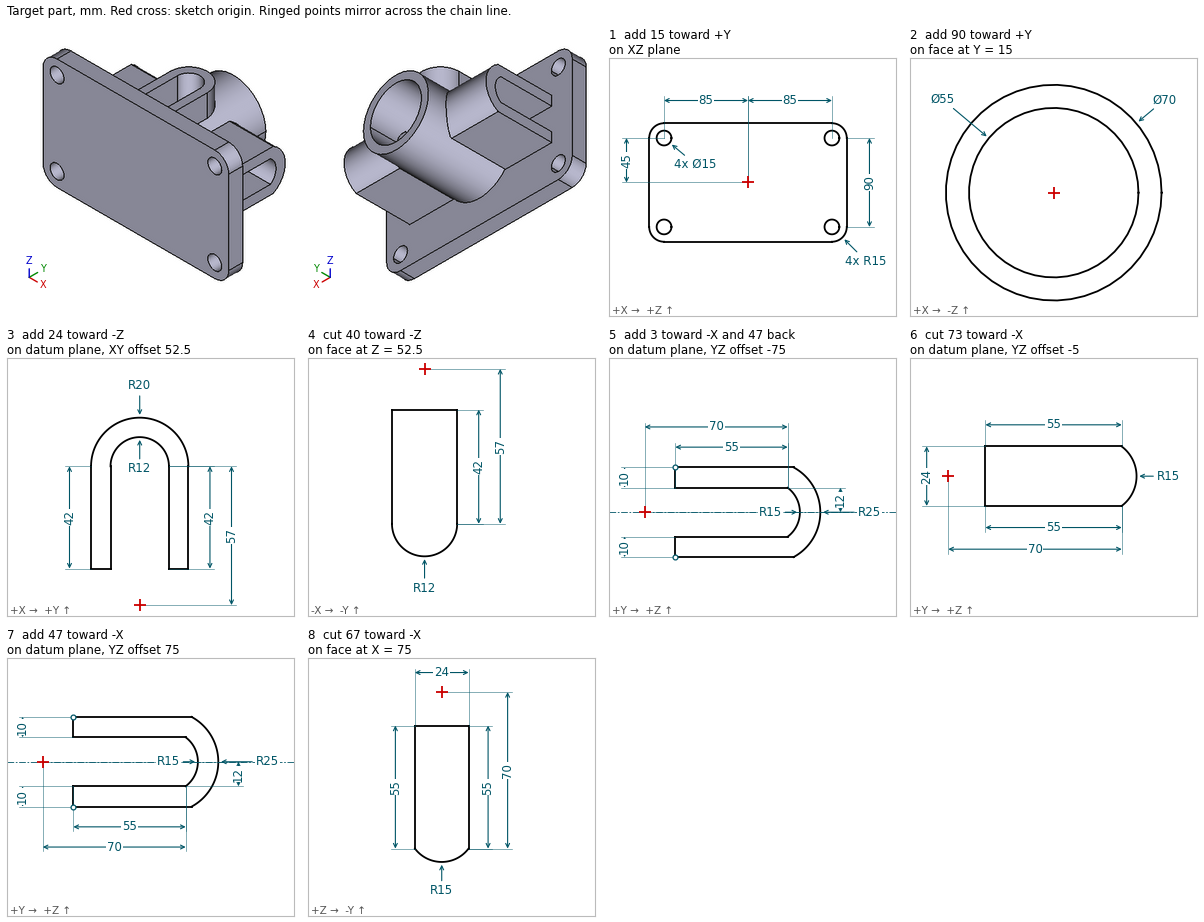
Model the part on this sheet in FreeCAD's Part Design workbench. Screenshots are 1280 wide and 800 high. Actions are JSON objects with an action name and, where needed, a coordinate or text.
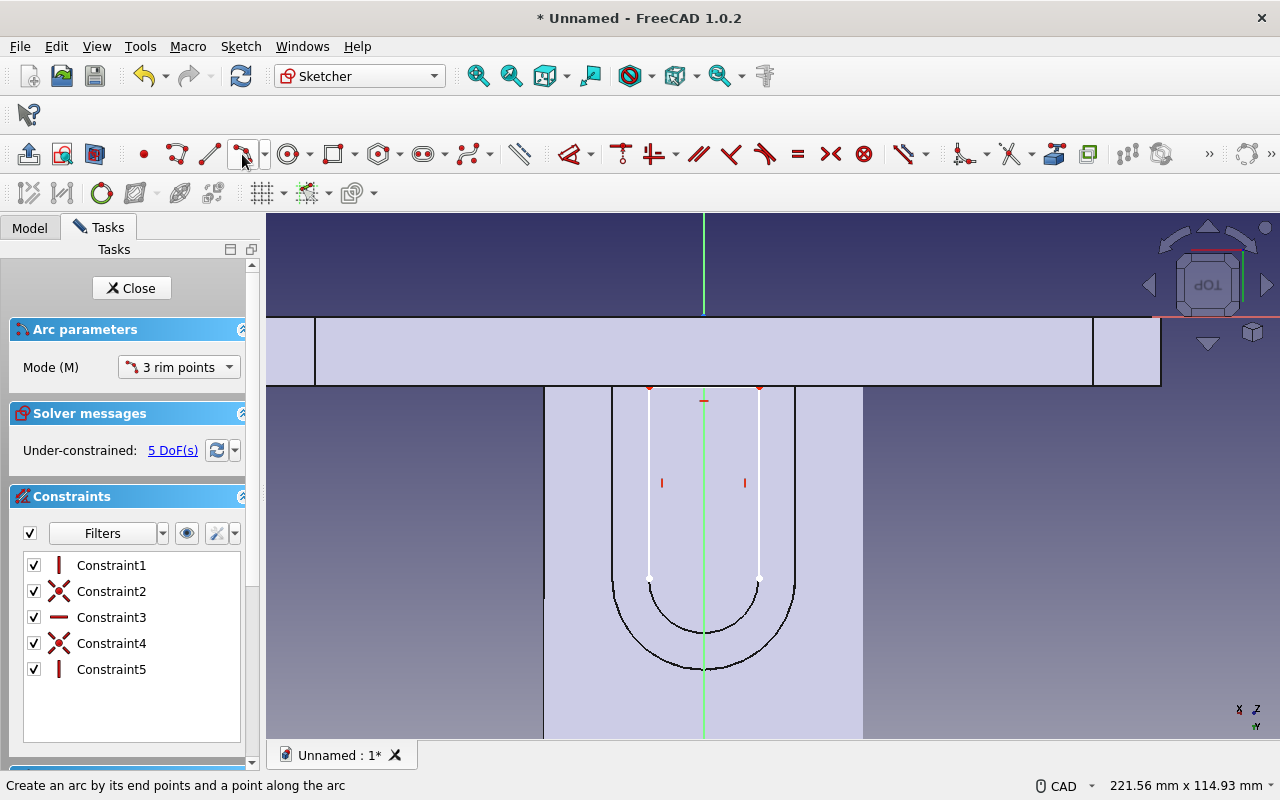
{"action": "left_click", "coordinate": [649, 579]}
{"action": "left_click", "coordinate": [759, 579]}
{"action": "left_click", "coordinate": [687, 630]}
{"action": "key", "text": "Escape"}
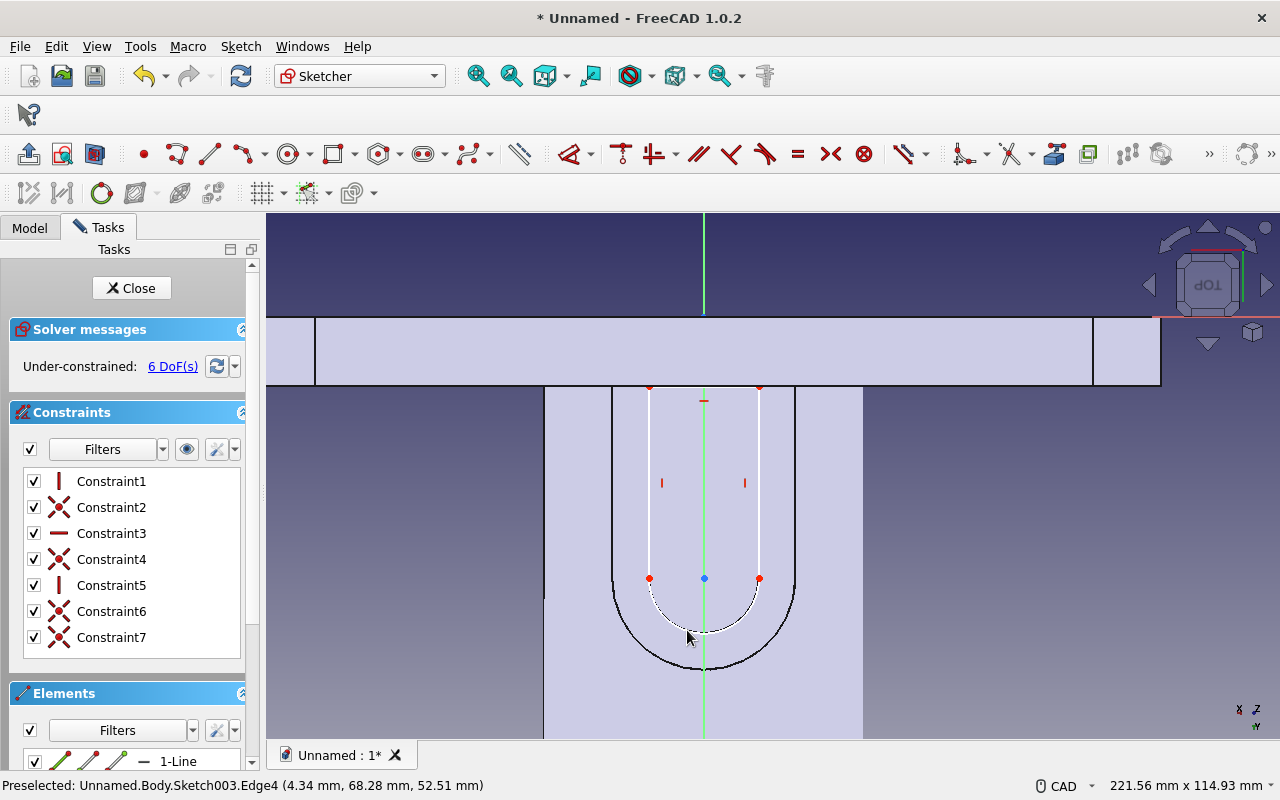
{"action": "left_click", "coordinate": [759, 521]}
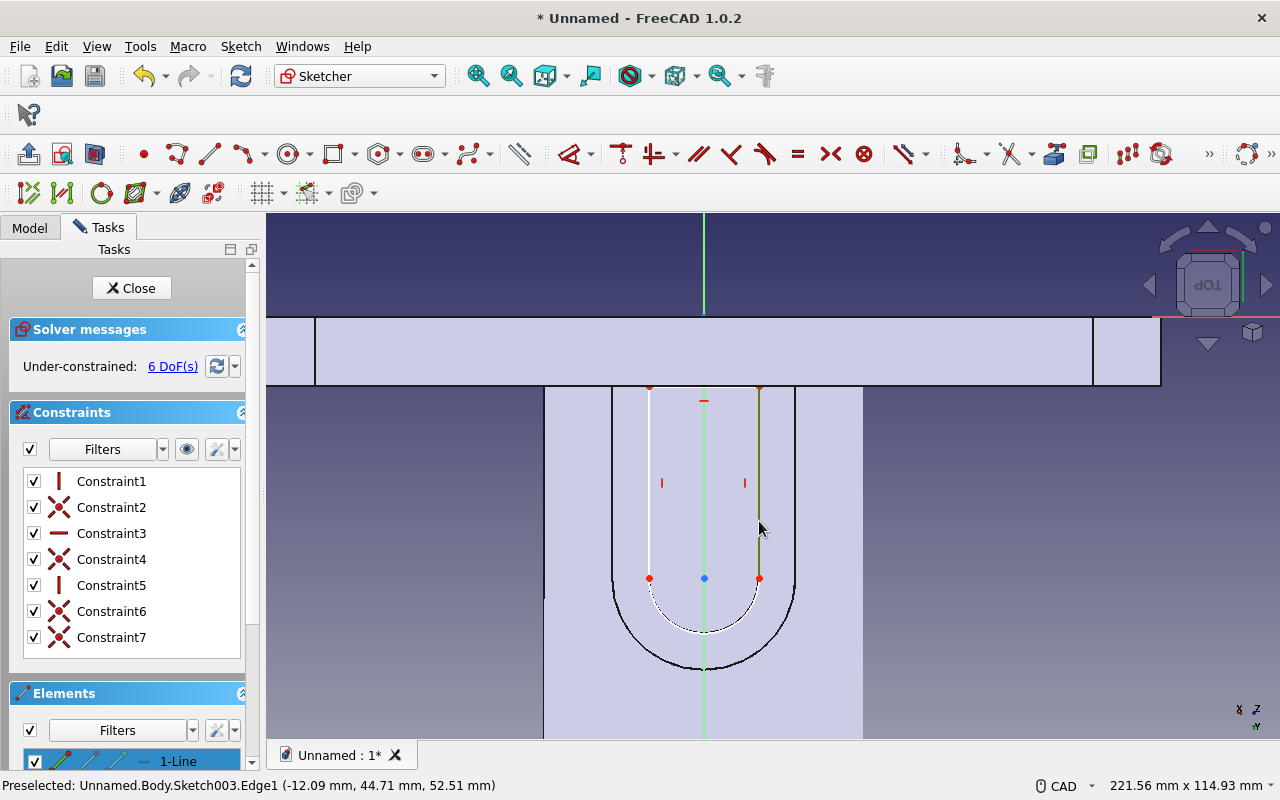
{"action": "left_click", "coordinate": [672, 623]}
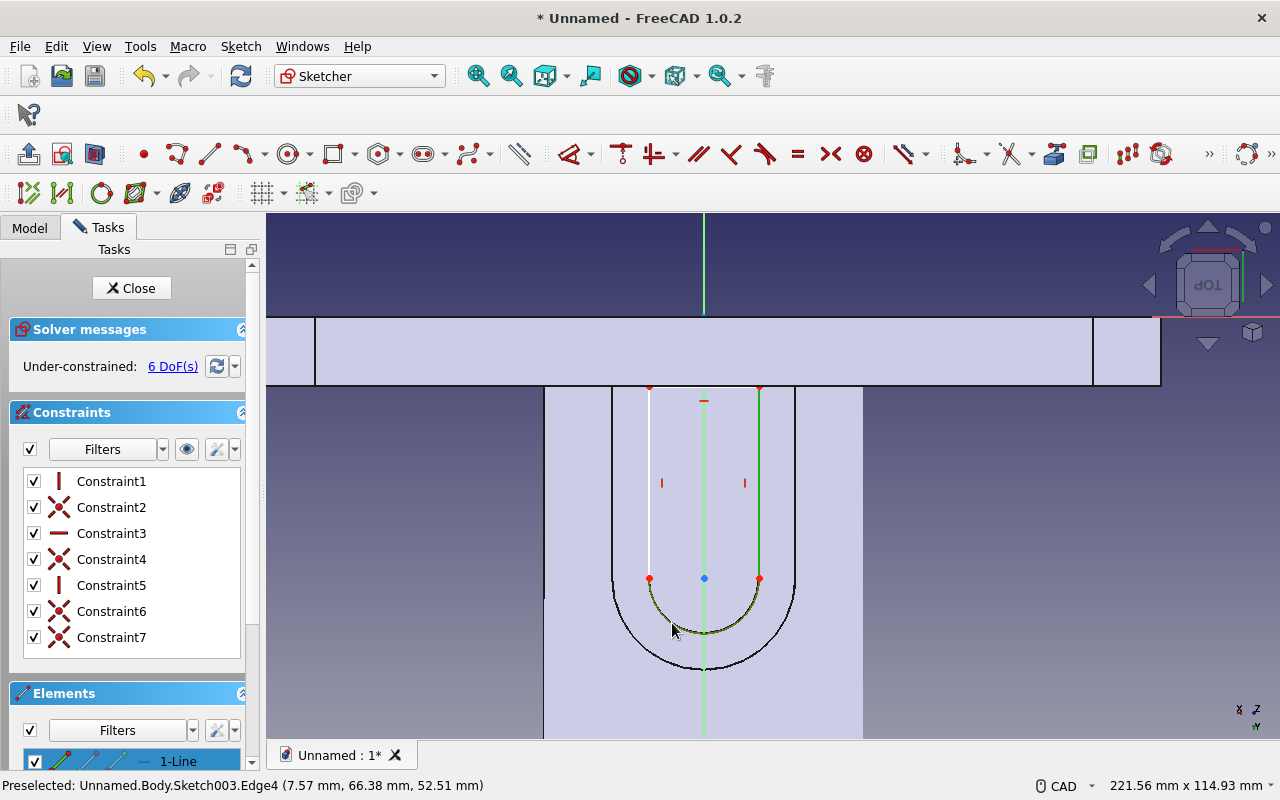
{"action": "key", "text": "t"}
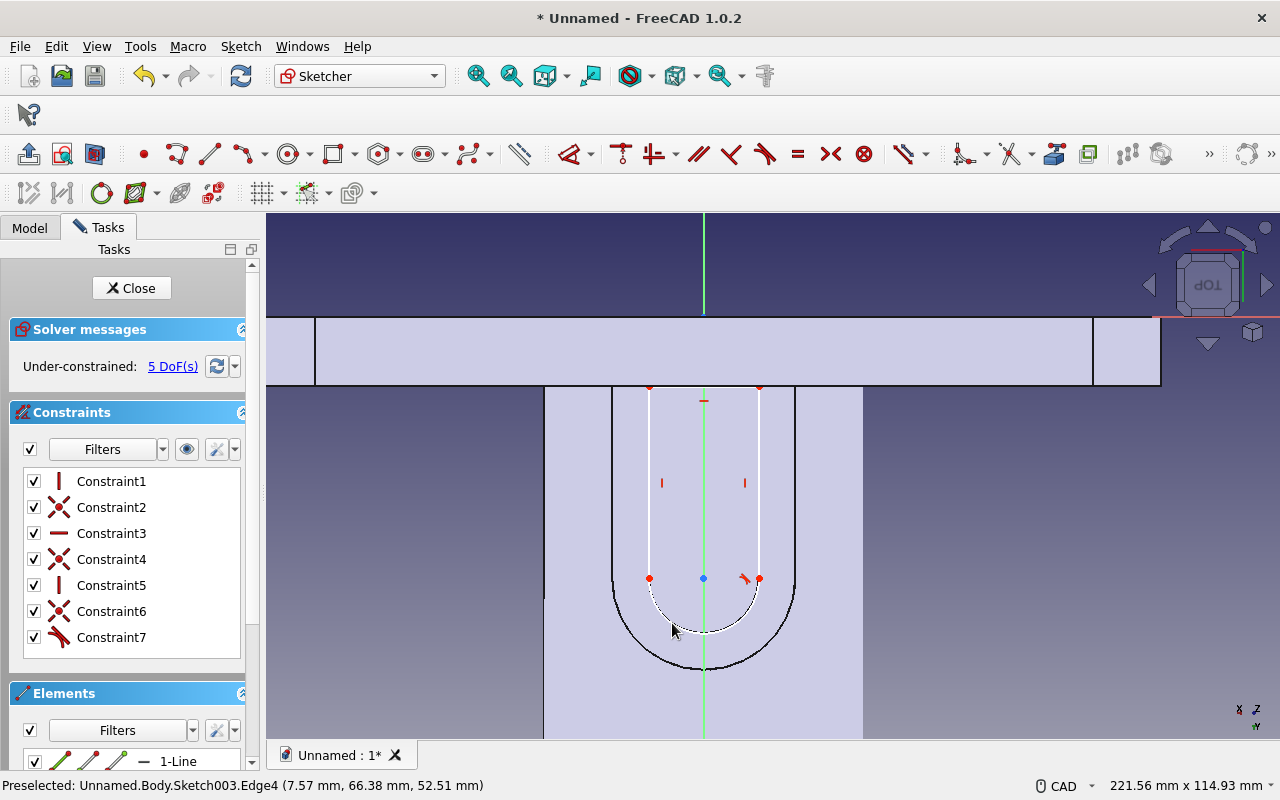
{"action": "left_click", "coordinate": [649, 445]}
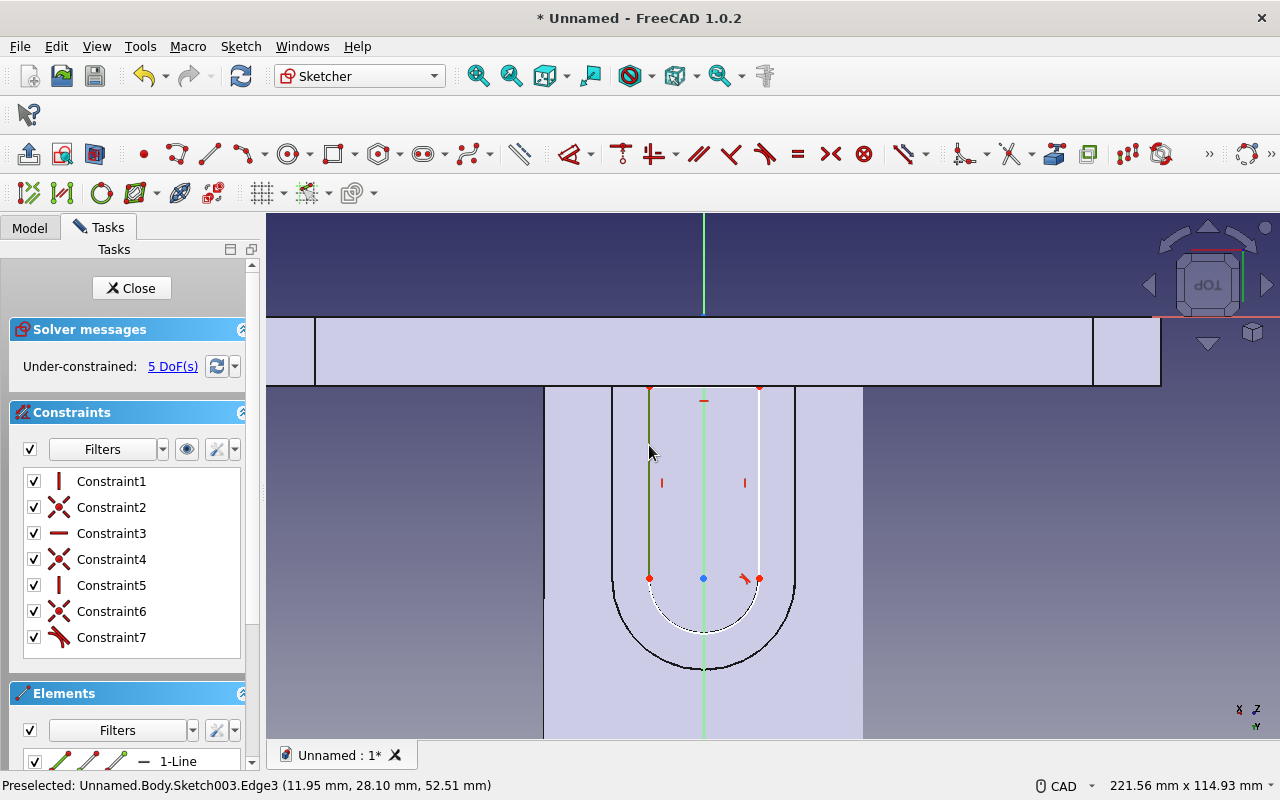
{"action": "left_click", "coordinate": [672, 623]}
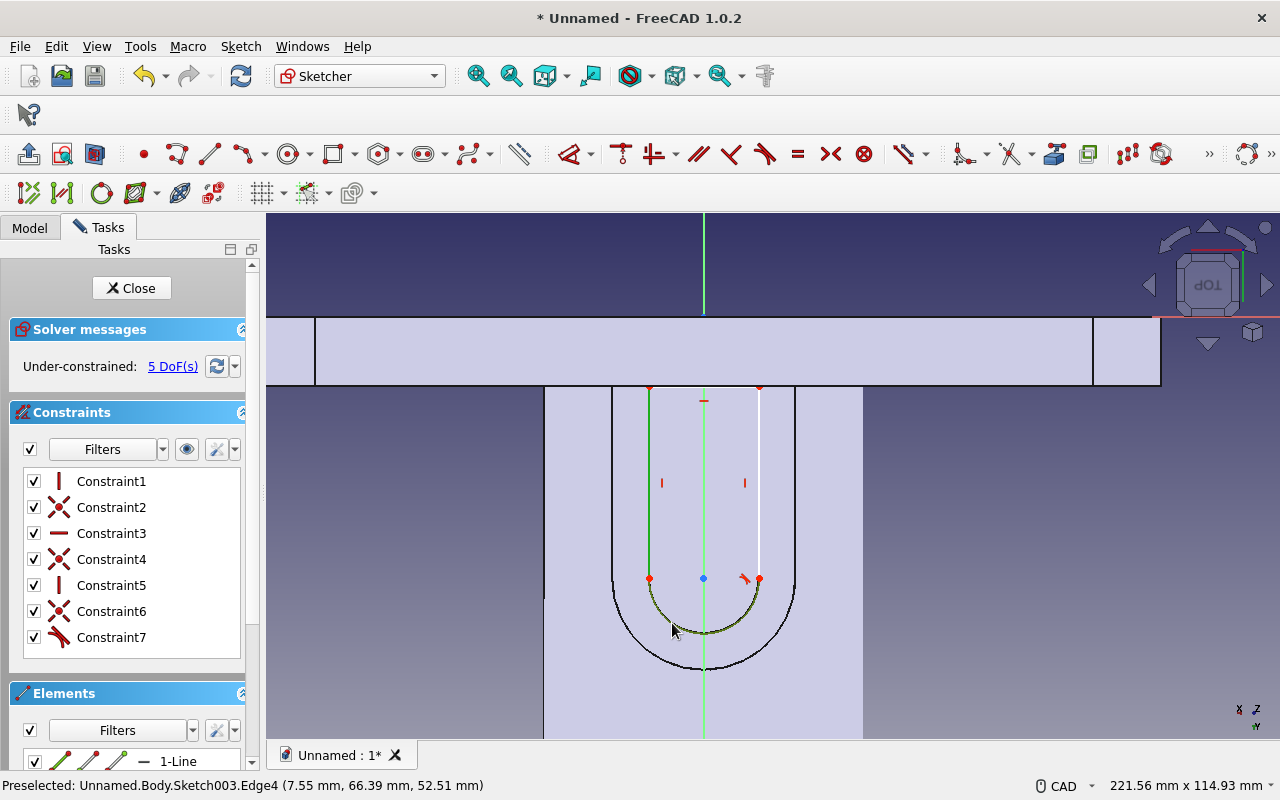
{"action": "left_click", "coordinate": [765, 154]}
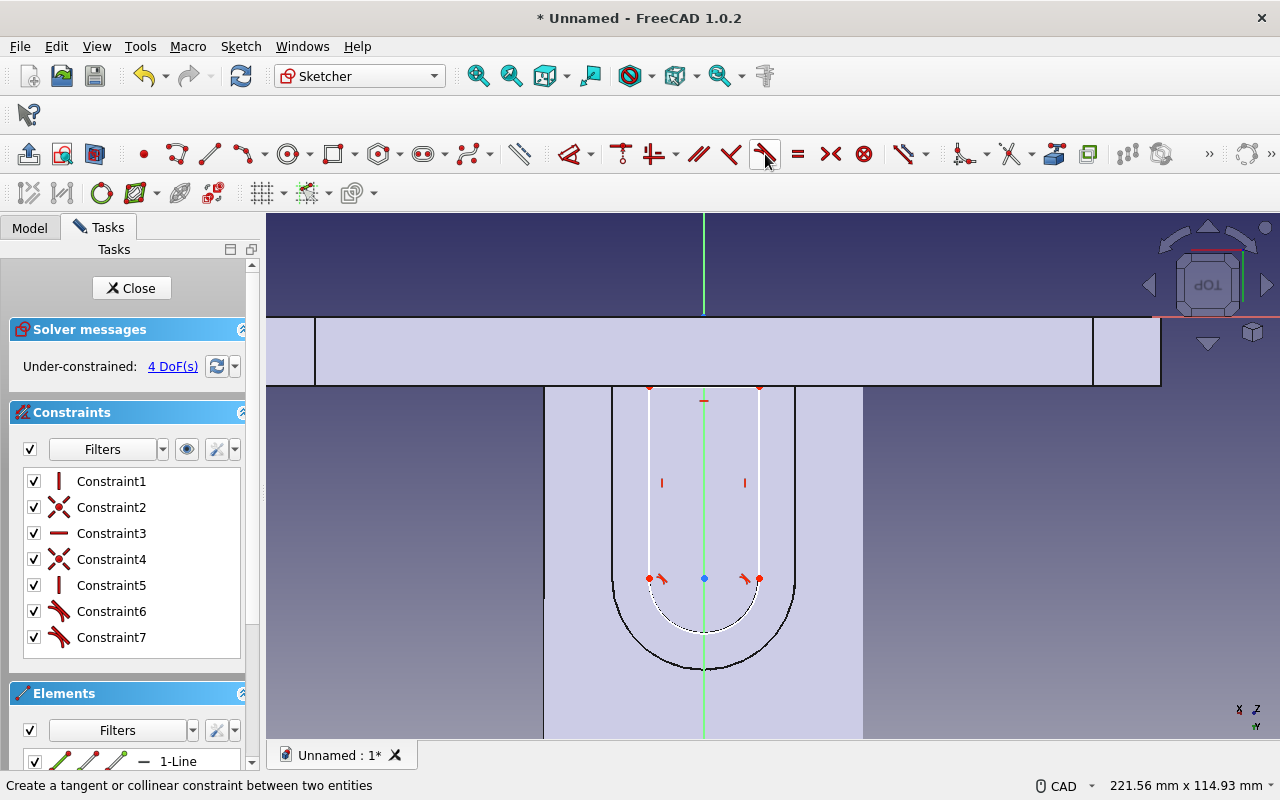
{"action": "left_click", "coordinate": [704, 579]}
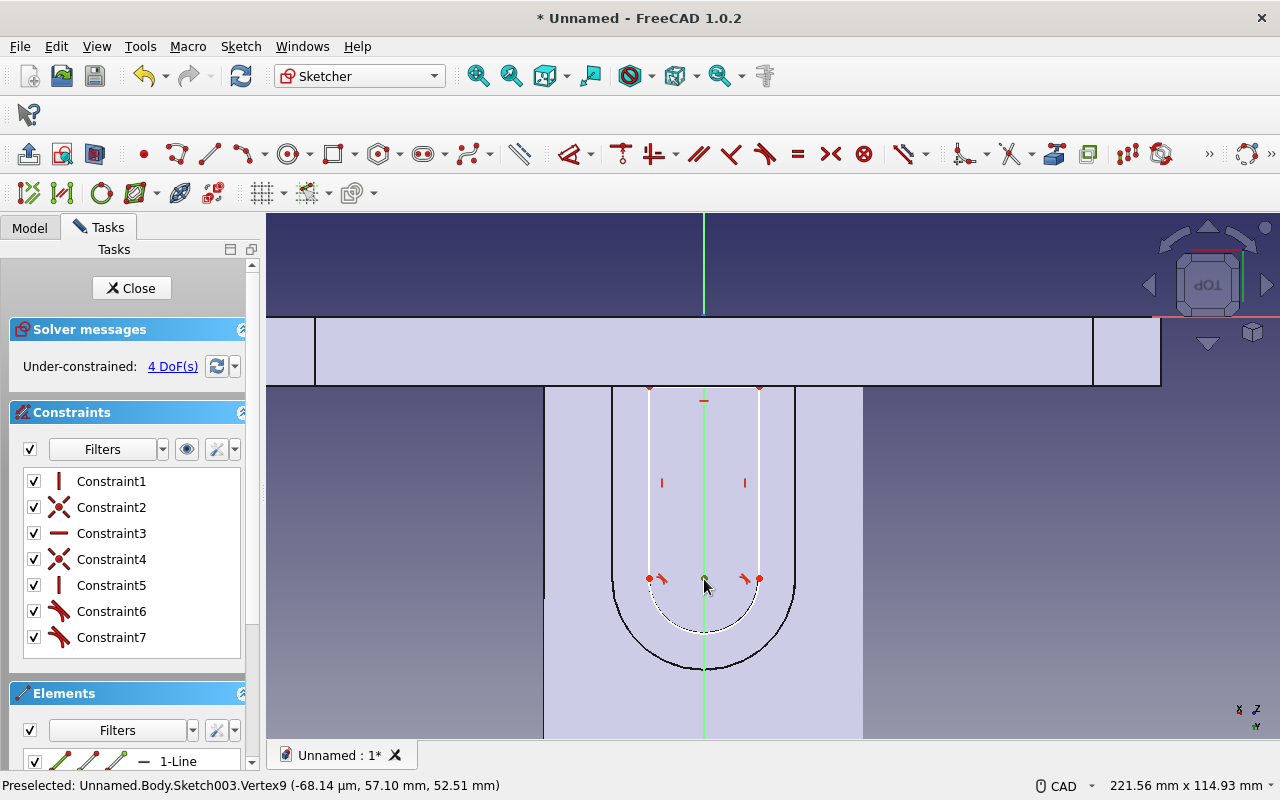
{"action": "left_click", "coordinate": [704, 677]}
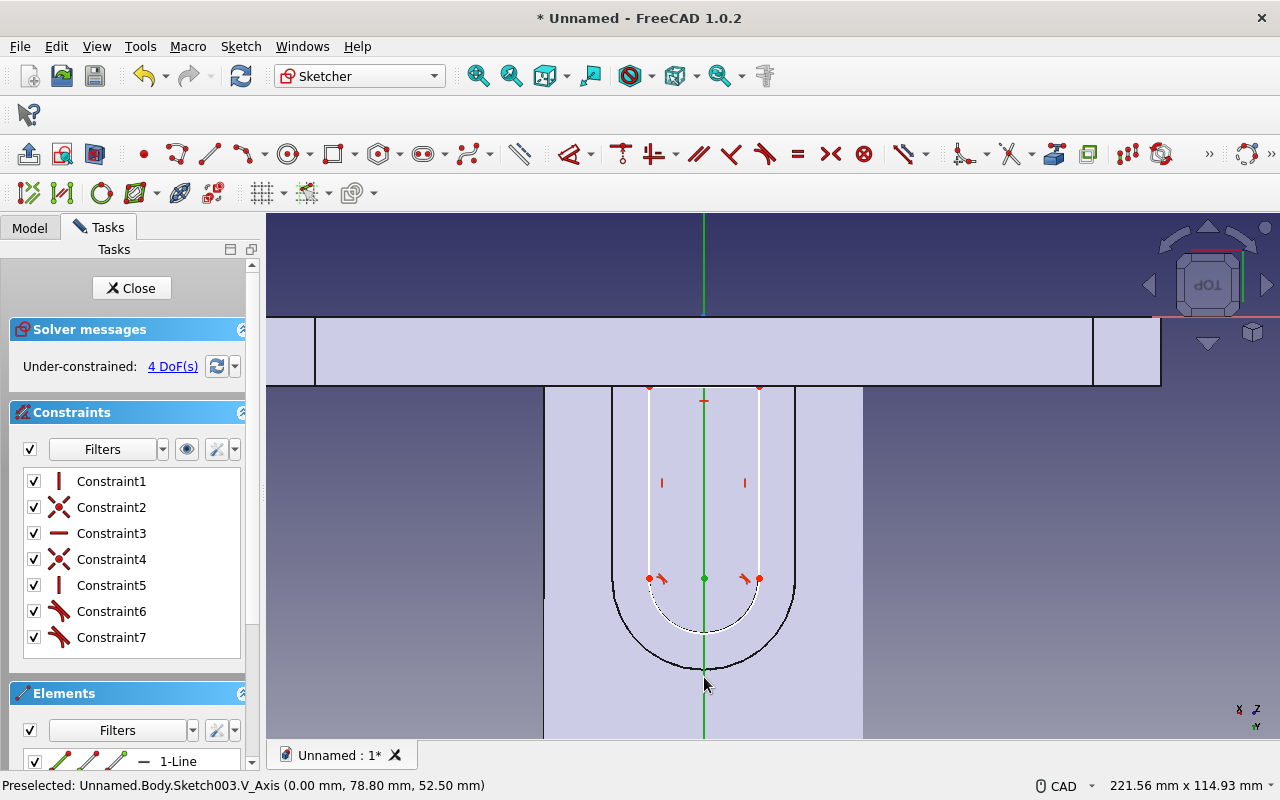
{"action": "left_click", "coordinate": [621, 154]}